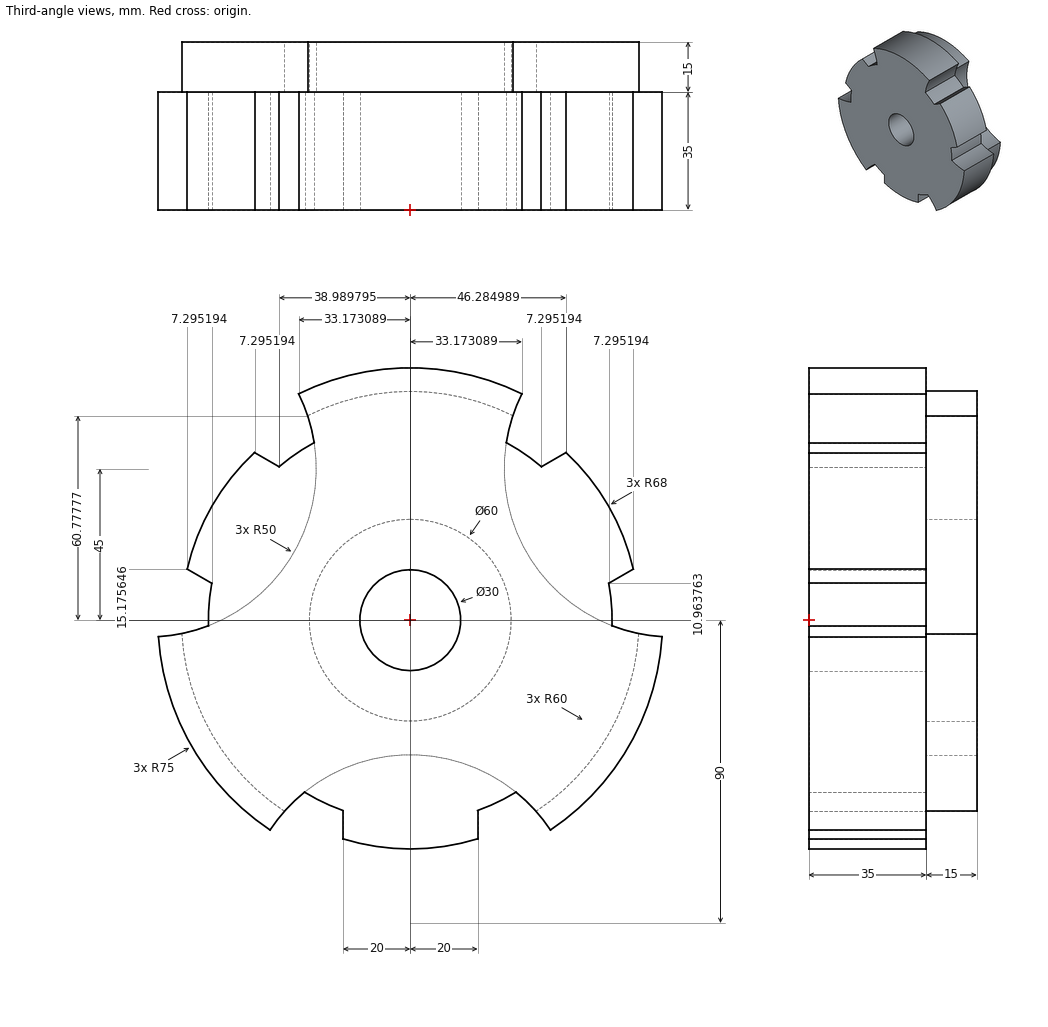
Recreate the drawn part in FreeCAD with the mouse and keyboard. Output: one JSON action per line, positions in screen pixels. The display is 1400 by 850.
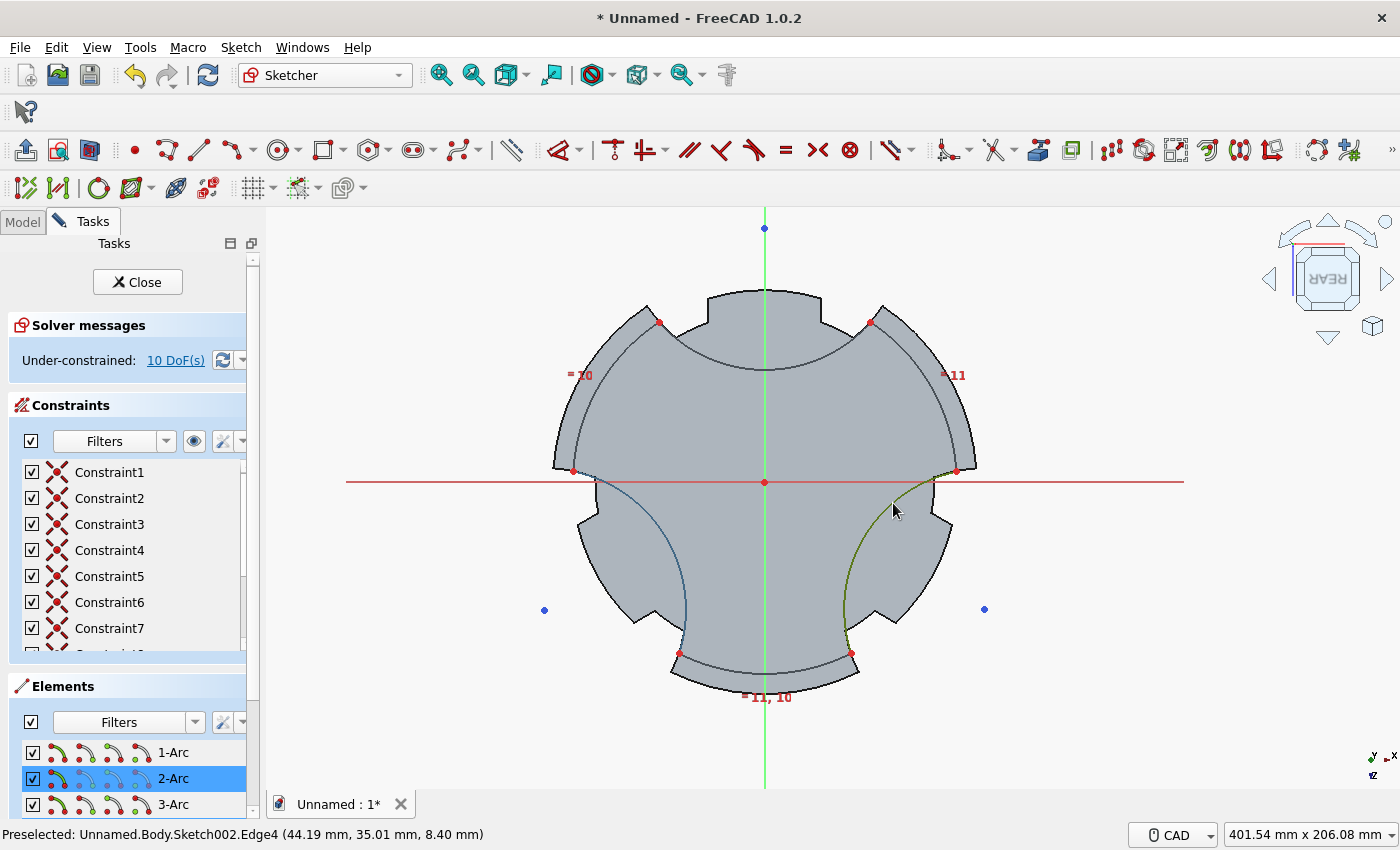
{"action": "left_click", "coordinate": [718, 362]}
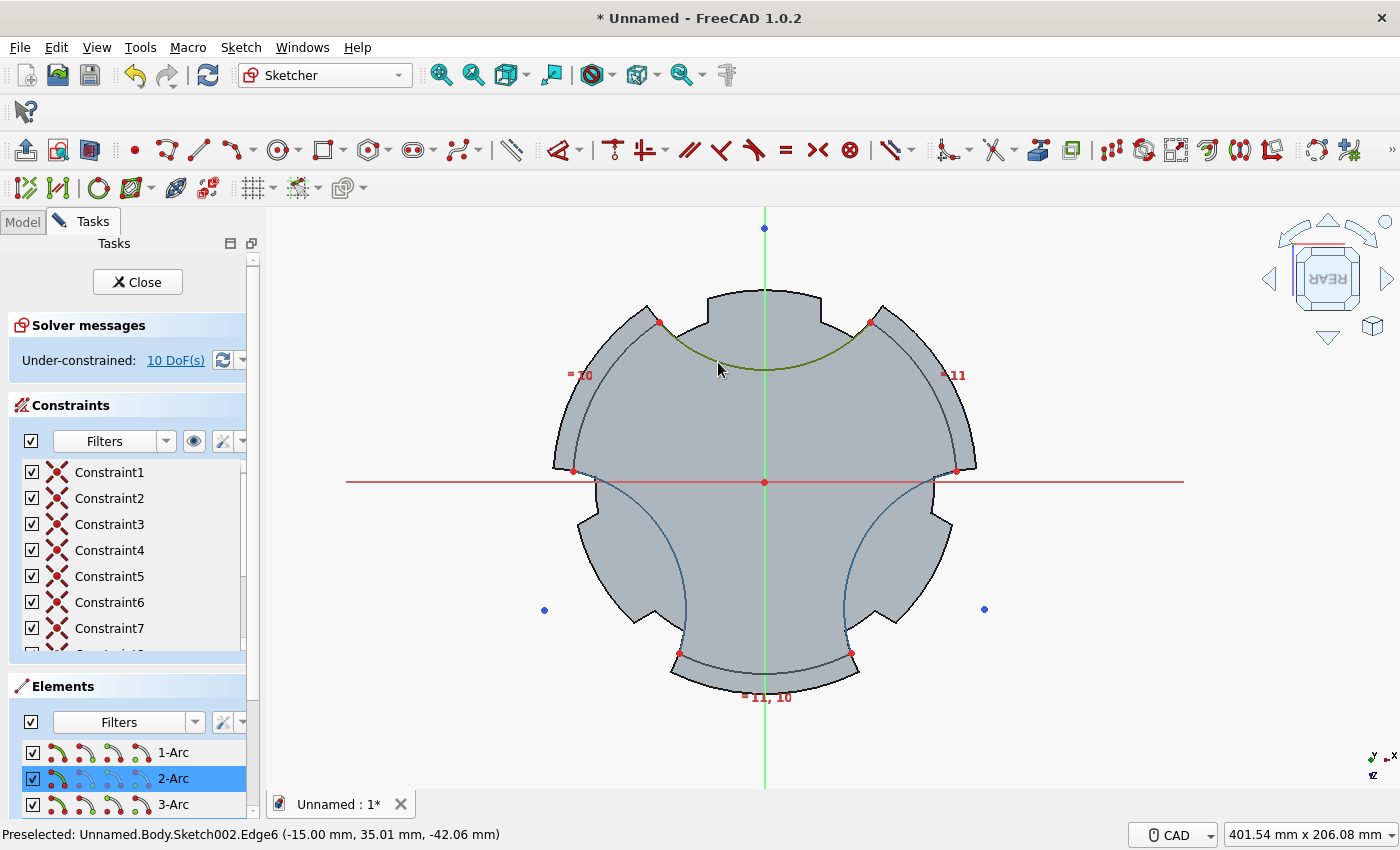
{"action": "left_click", "coordinate": [786, 150]}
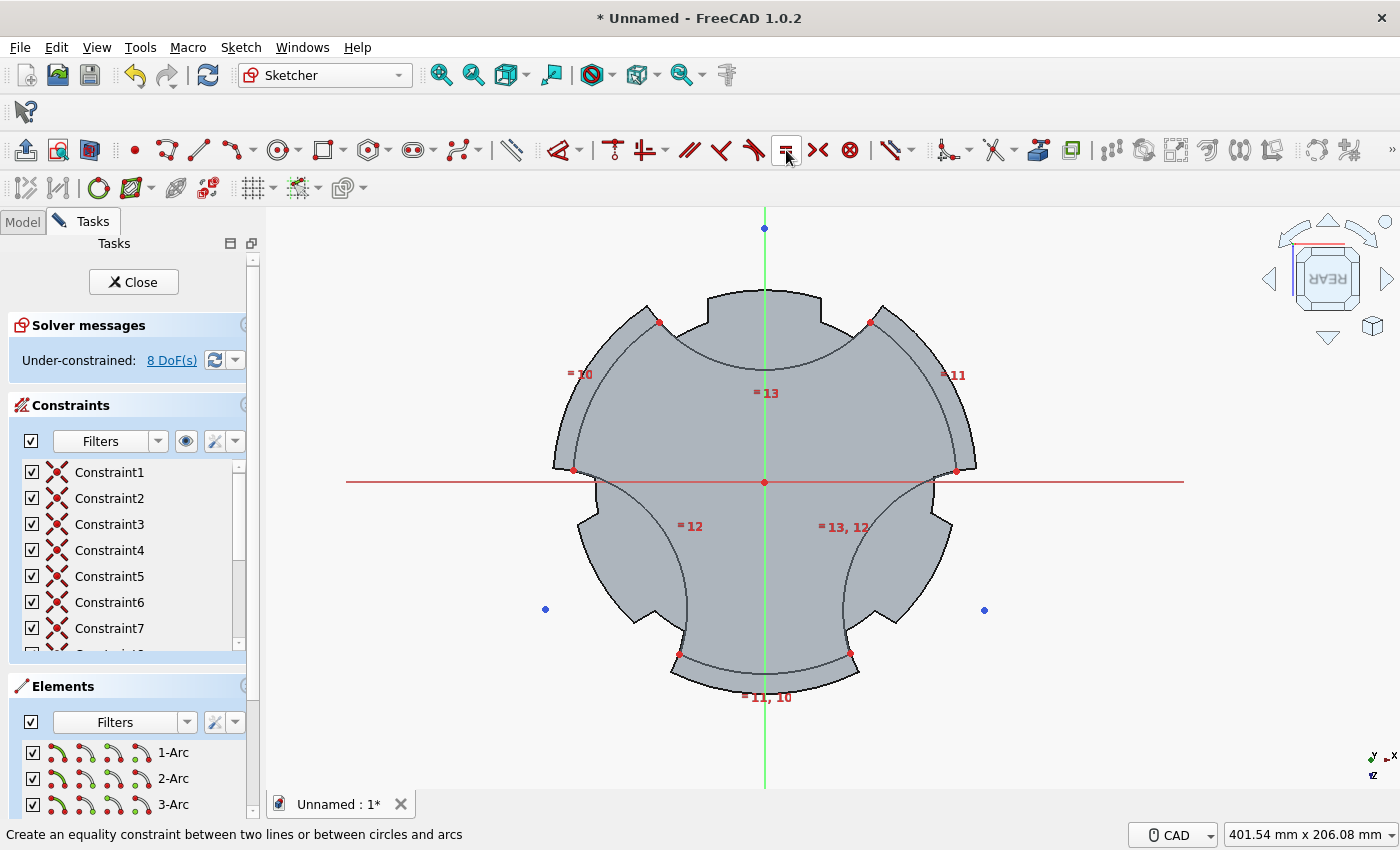
{"action": "scroll", "coordinate": [763, 709], "scroll_direction": "down", "scroll_amount": 1}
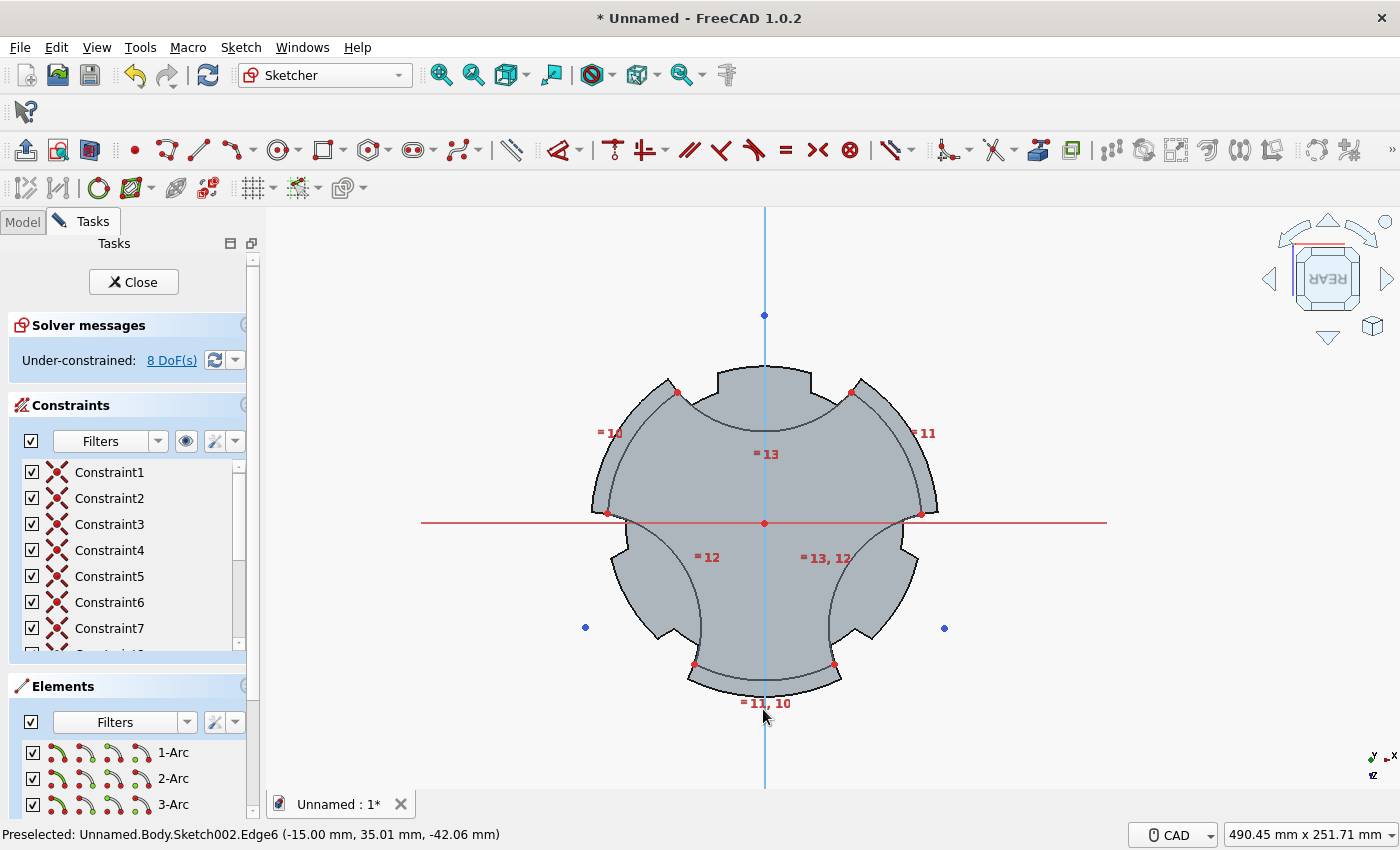
{"action": "left_click", "coordinate": [765, 316]}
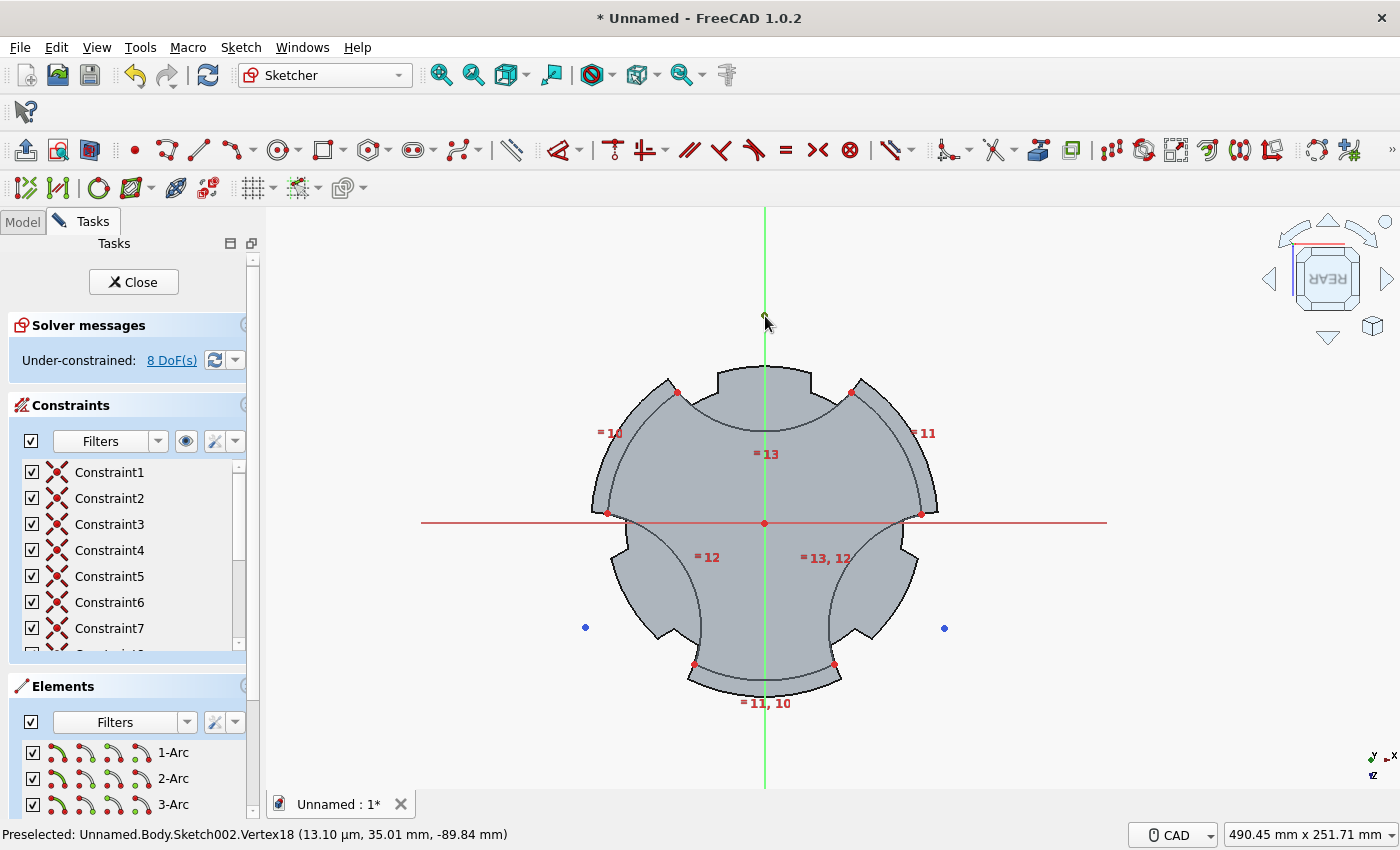
{"action": "left_click", "coordinate": [765, 723]}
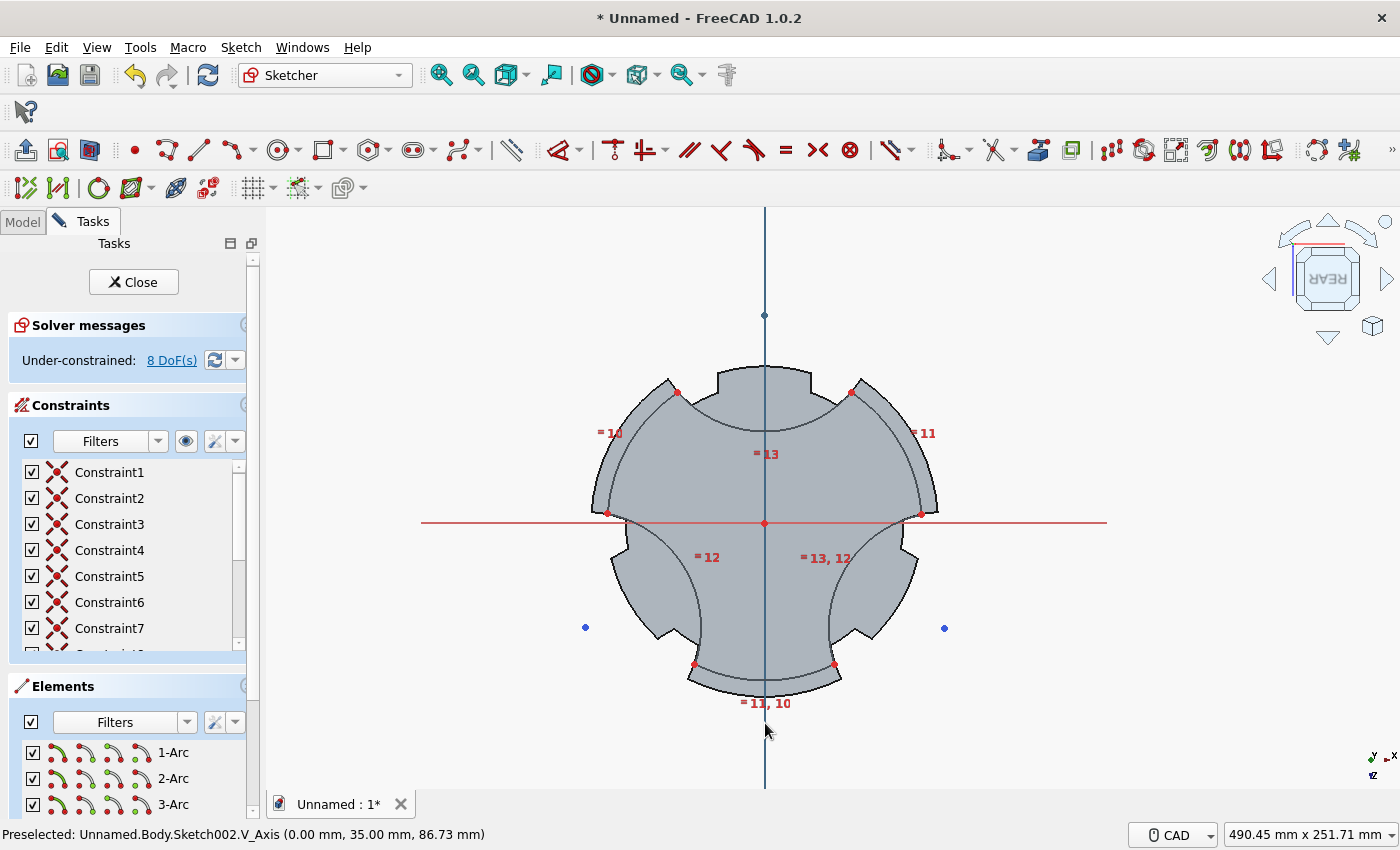
{"action": "left_click", "coordinate": [614, 150]}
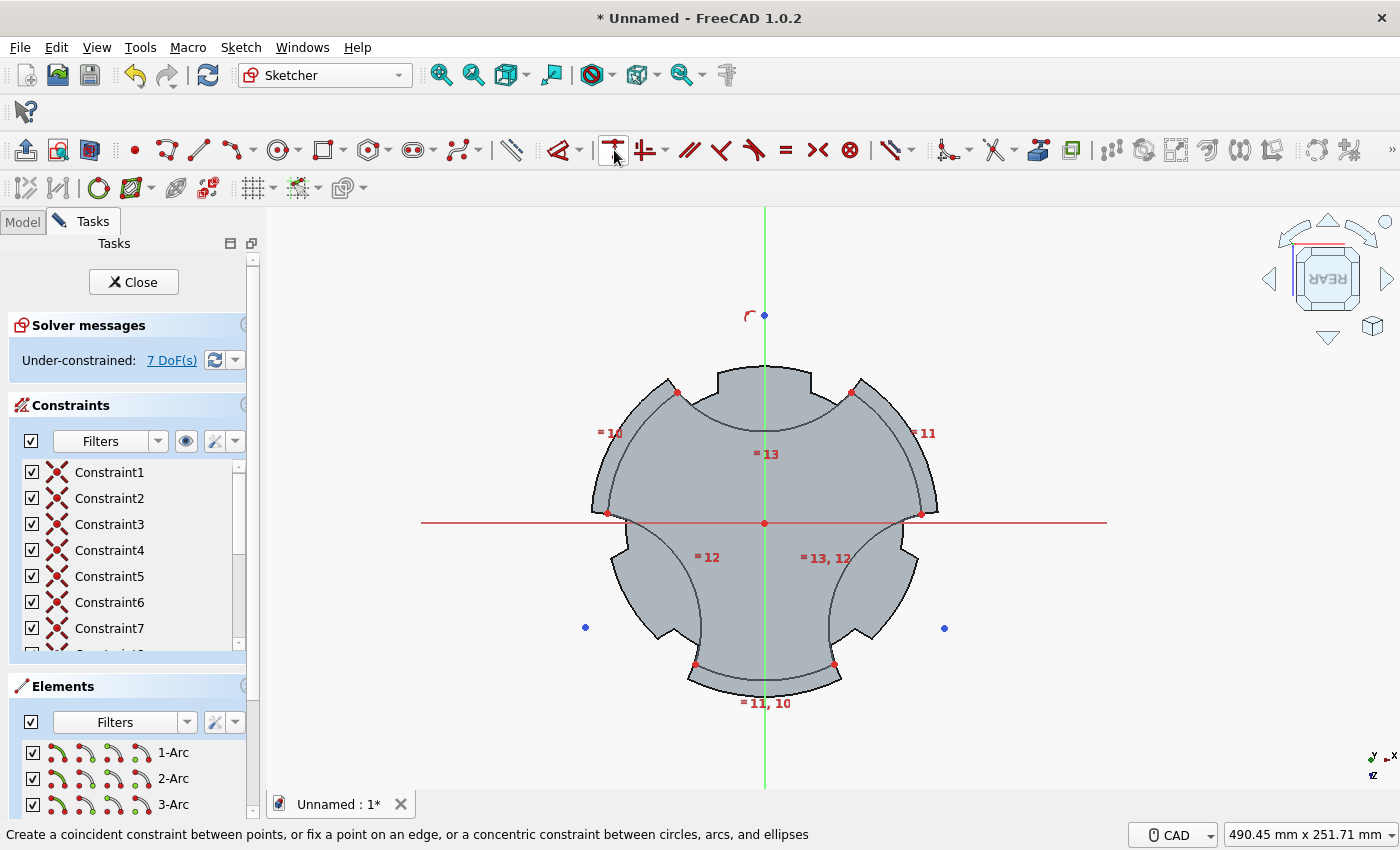
{"action": "left_click", "coordinate": [558, 150]}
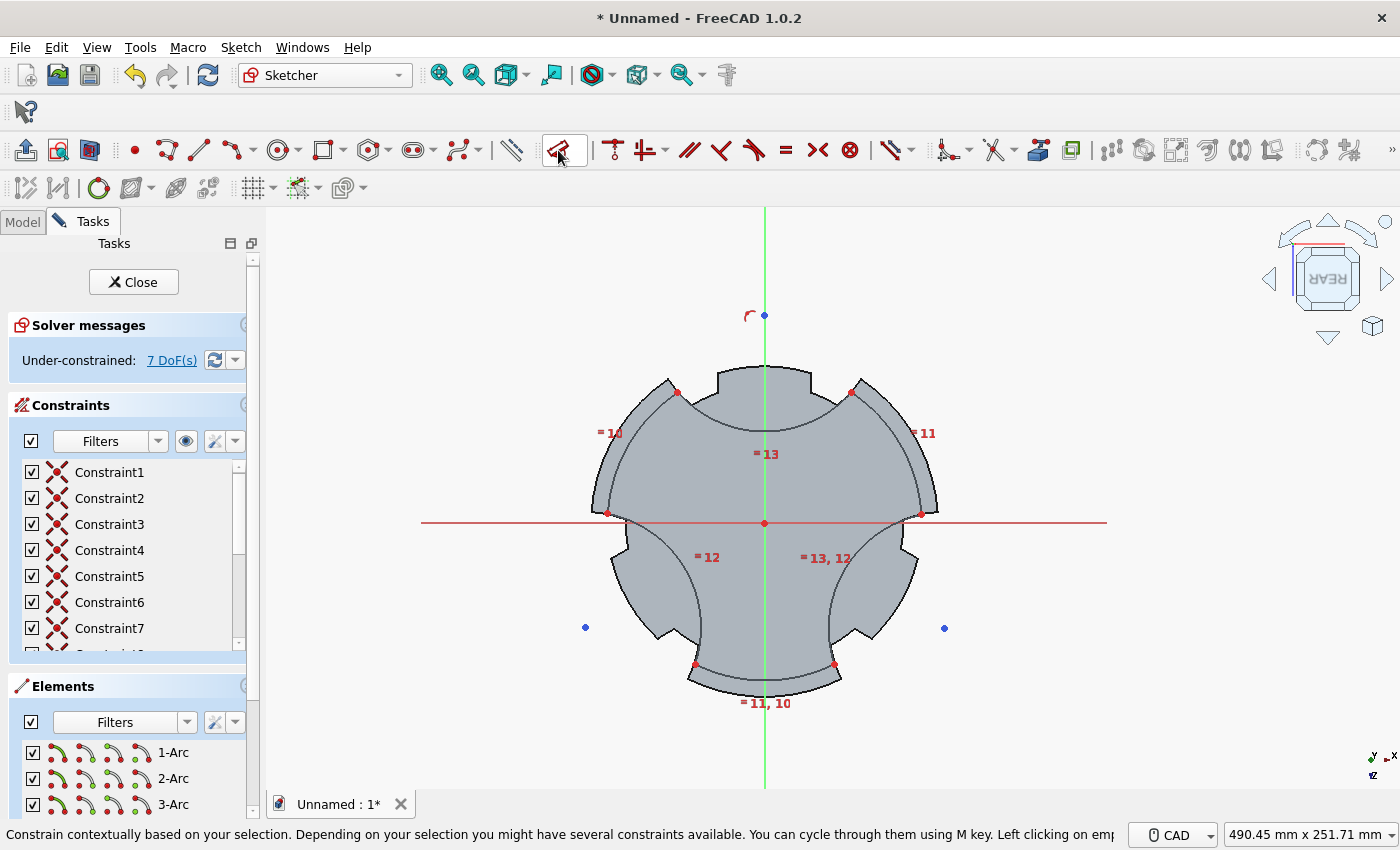
{"action": "left_click", "coordinate": [645, 421]}
{"action": "left_click", "coordinate": [621, 400]}